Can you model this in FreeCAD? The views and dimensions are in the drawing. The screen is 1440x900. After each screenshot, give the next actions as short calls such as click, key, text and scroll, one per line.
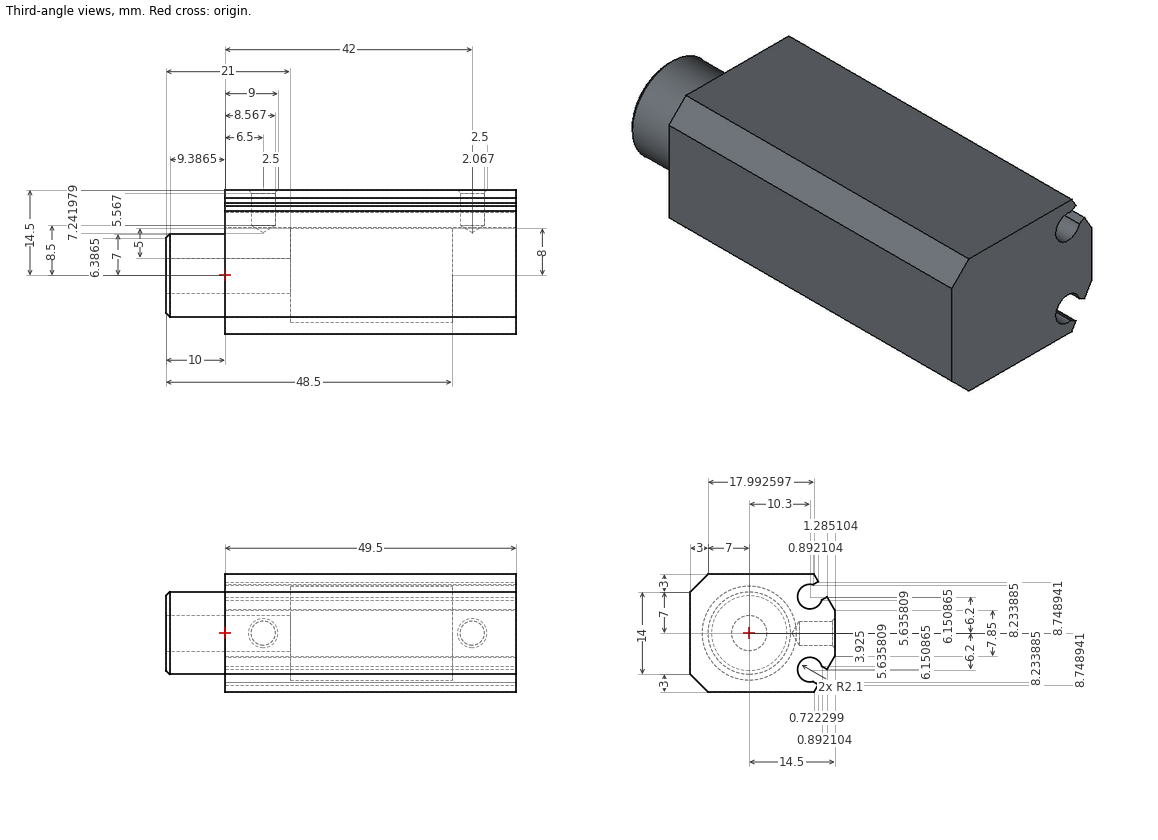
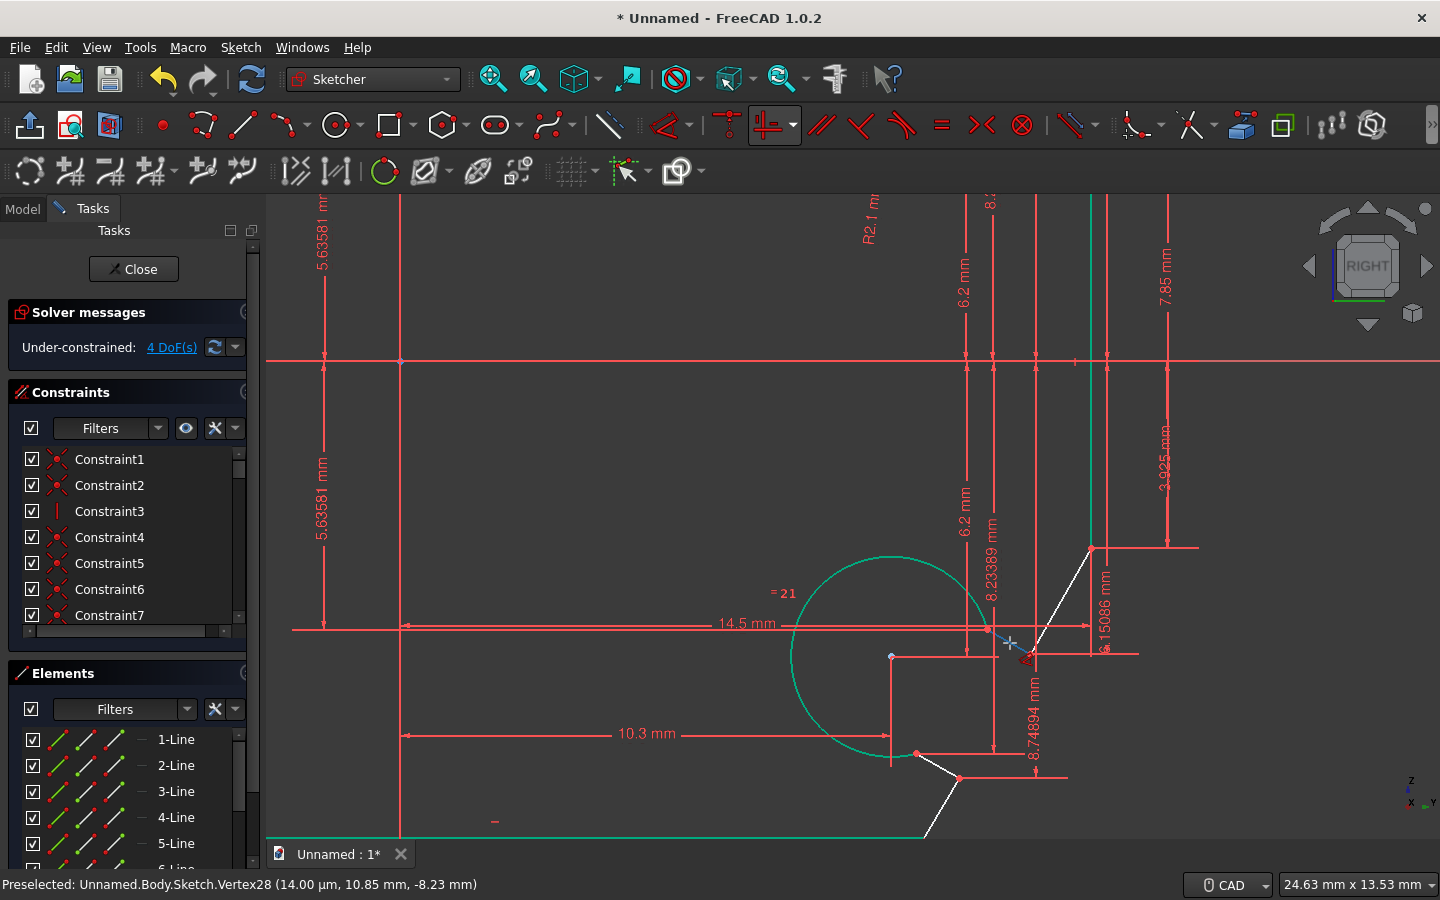
click(1009, 642)
click(1009, 688)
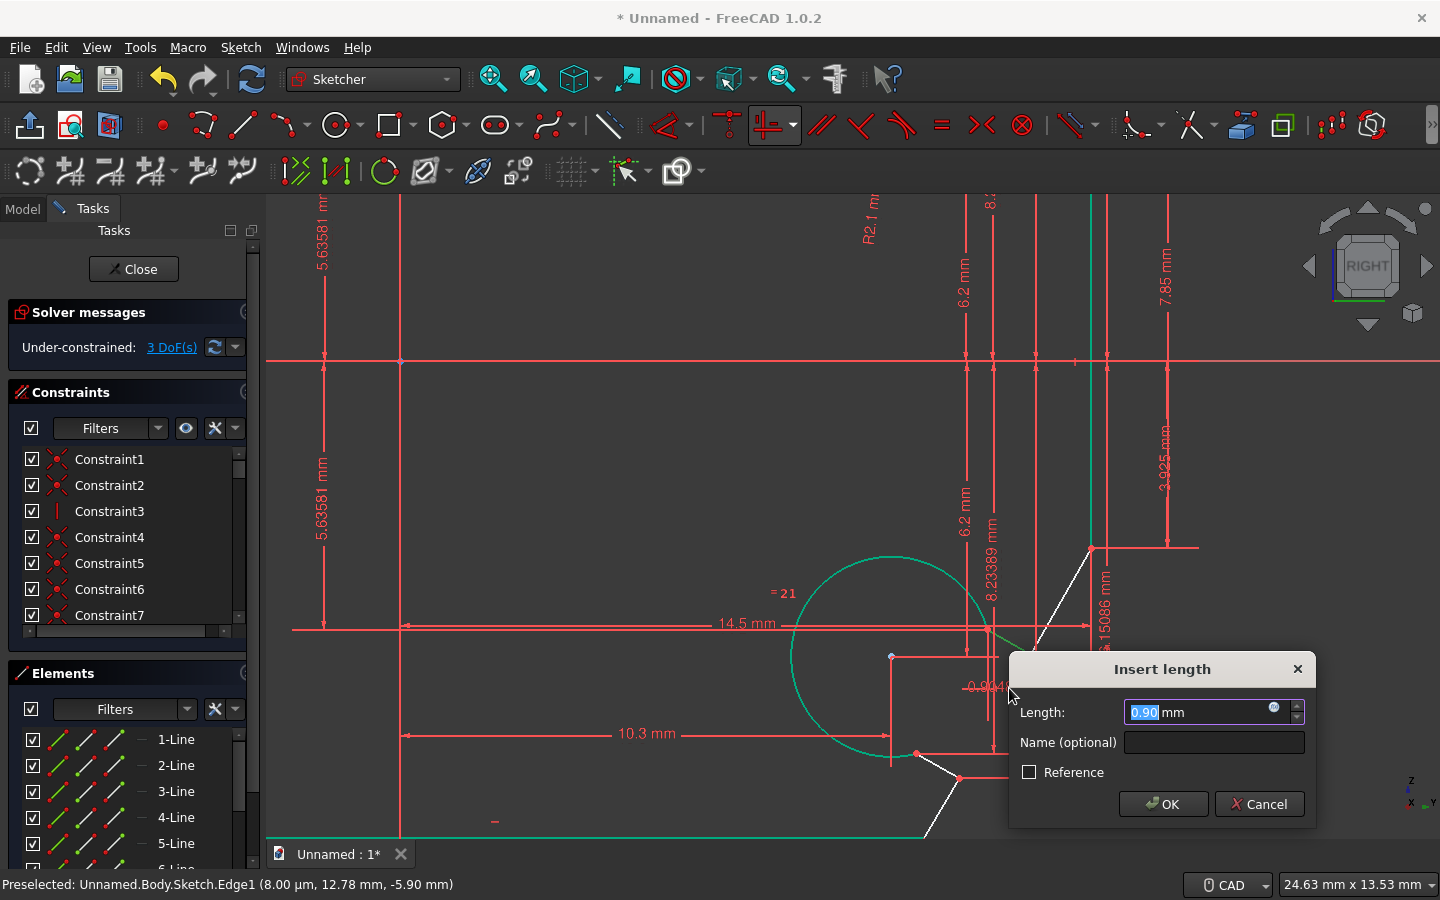
text(0.892104)
key(Return)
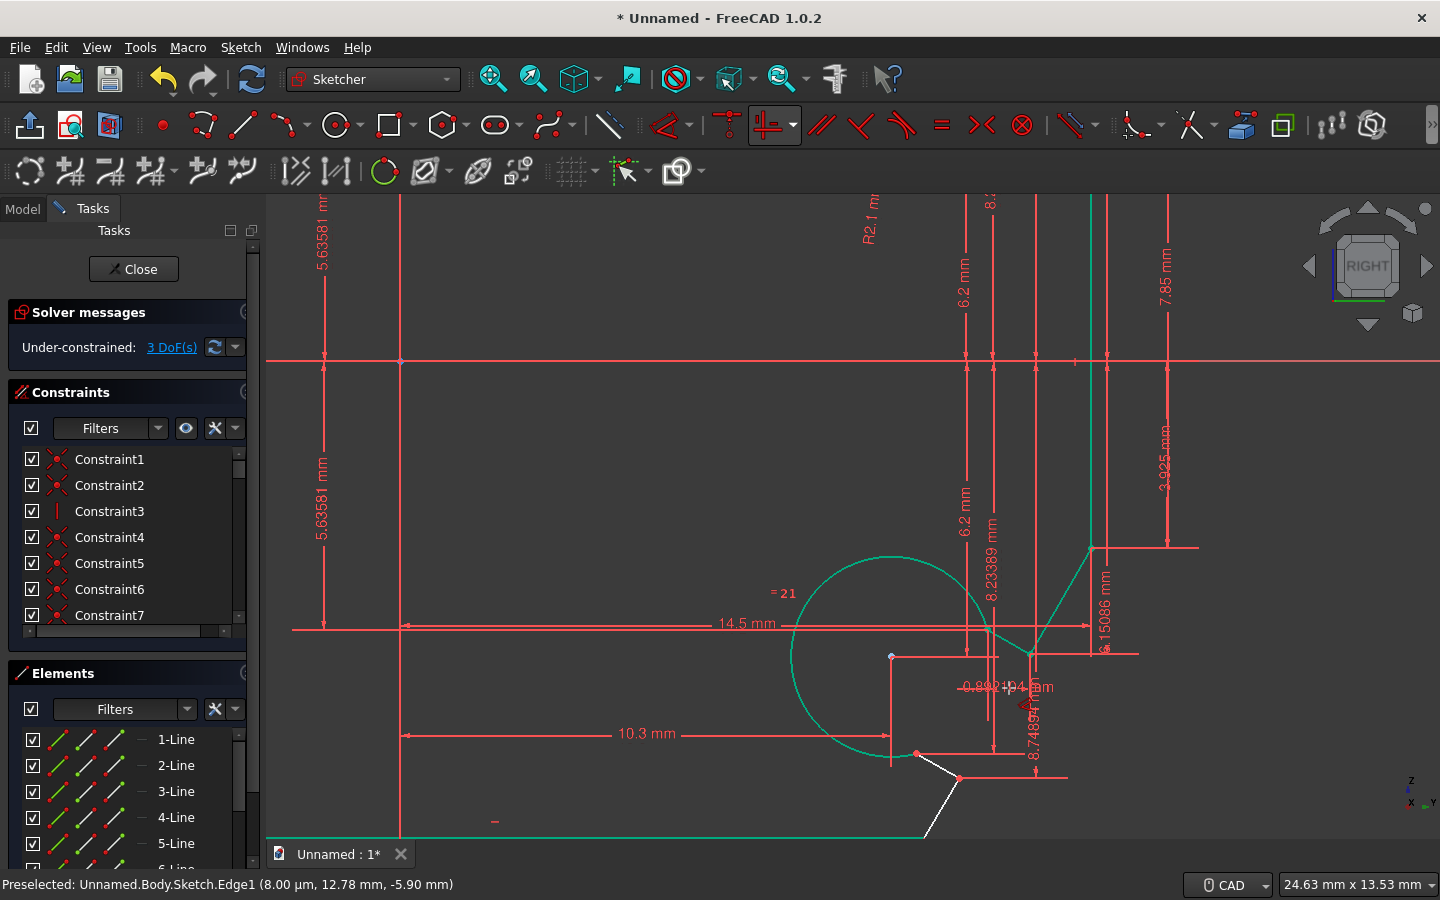
scroll(1010, 643, down, 4)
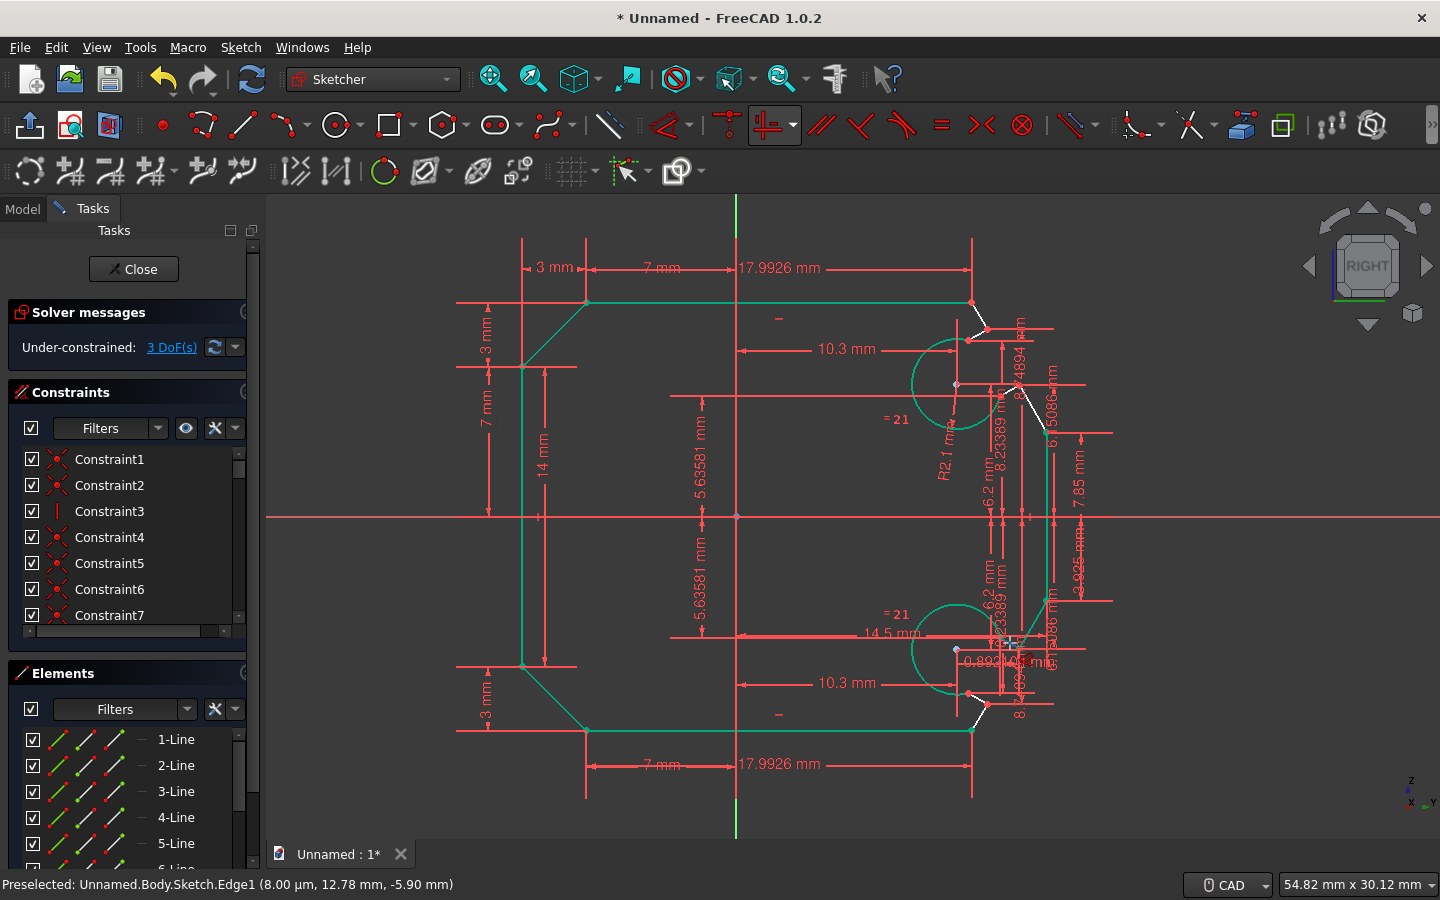
scroll(1039, 418, up, 2)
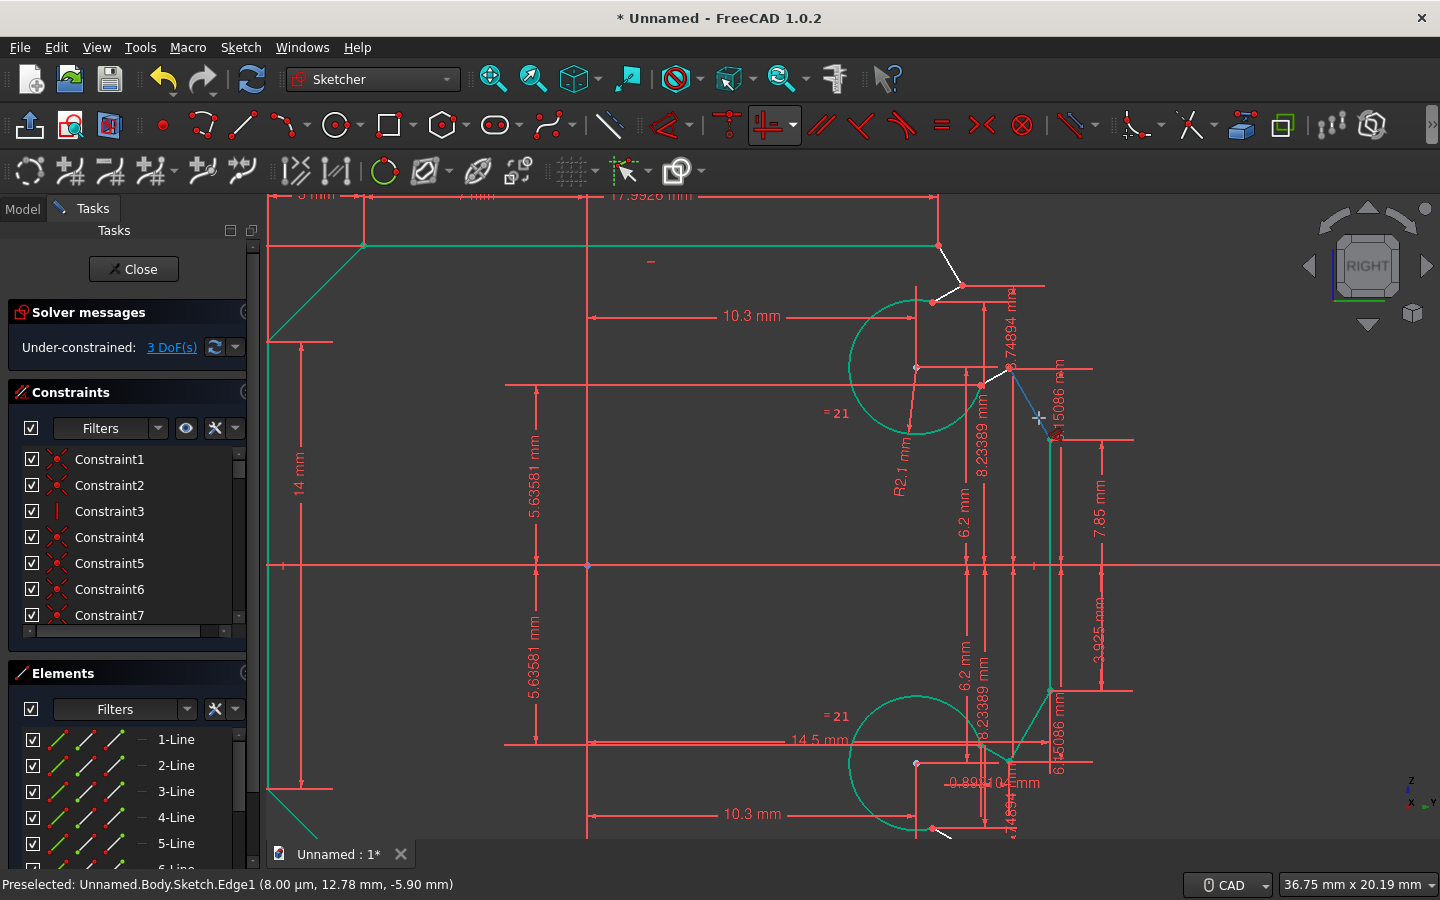
click(1038, 419)
click(1030, 474)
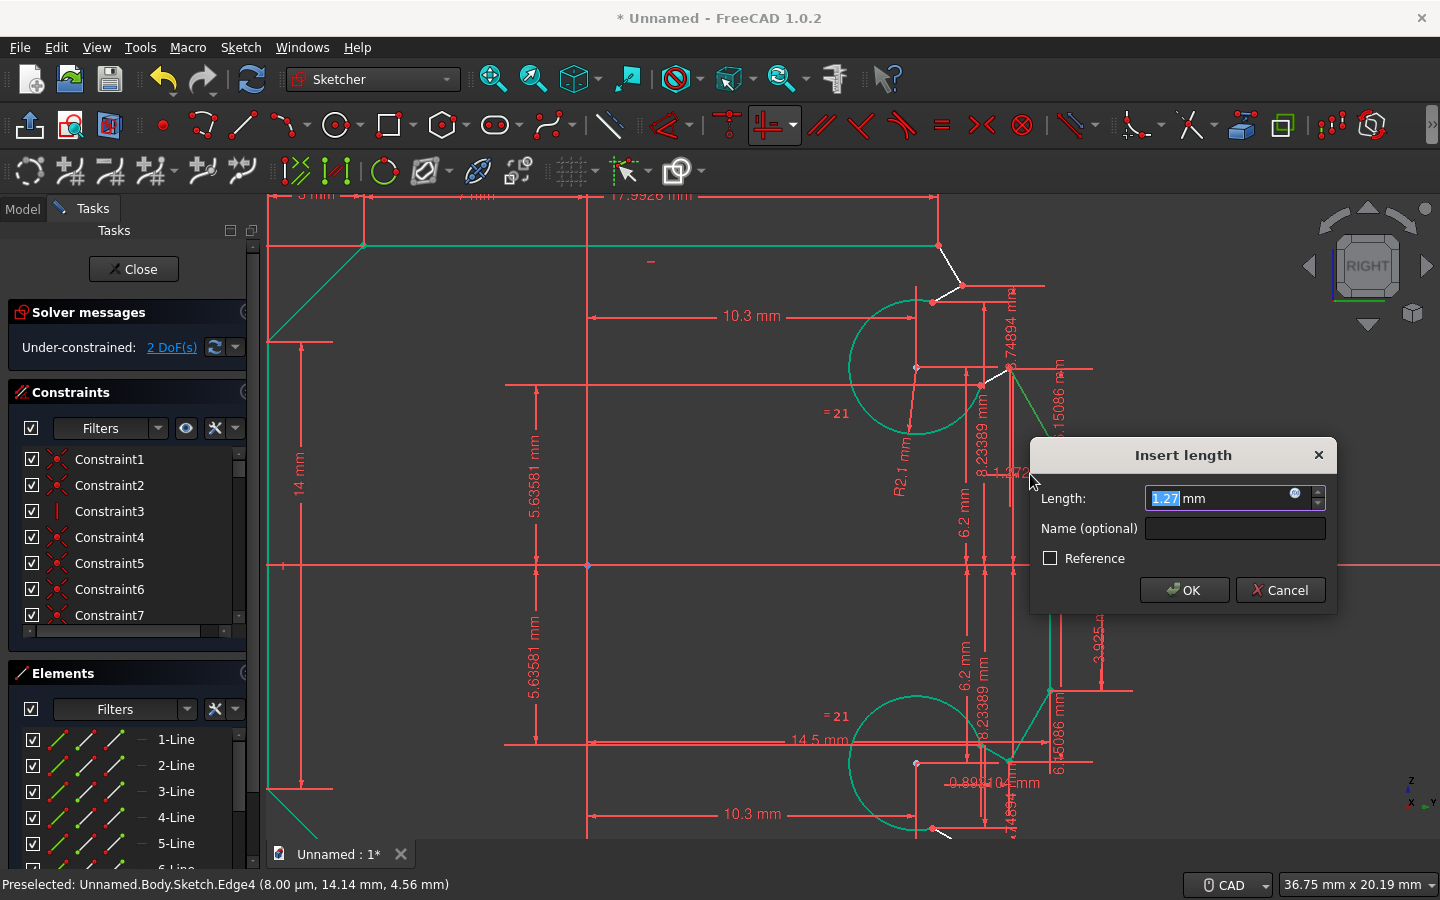
text(1.285104)
key(Return)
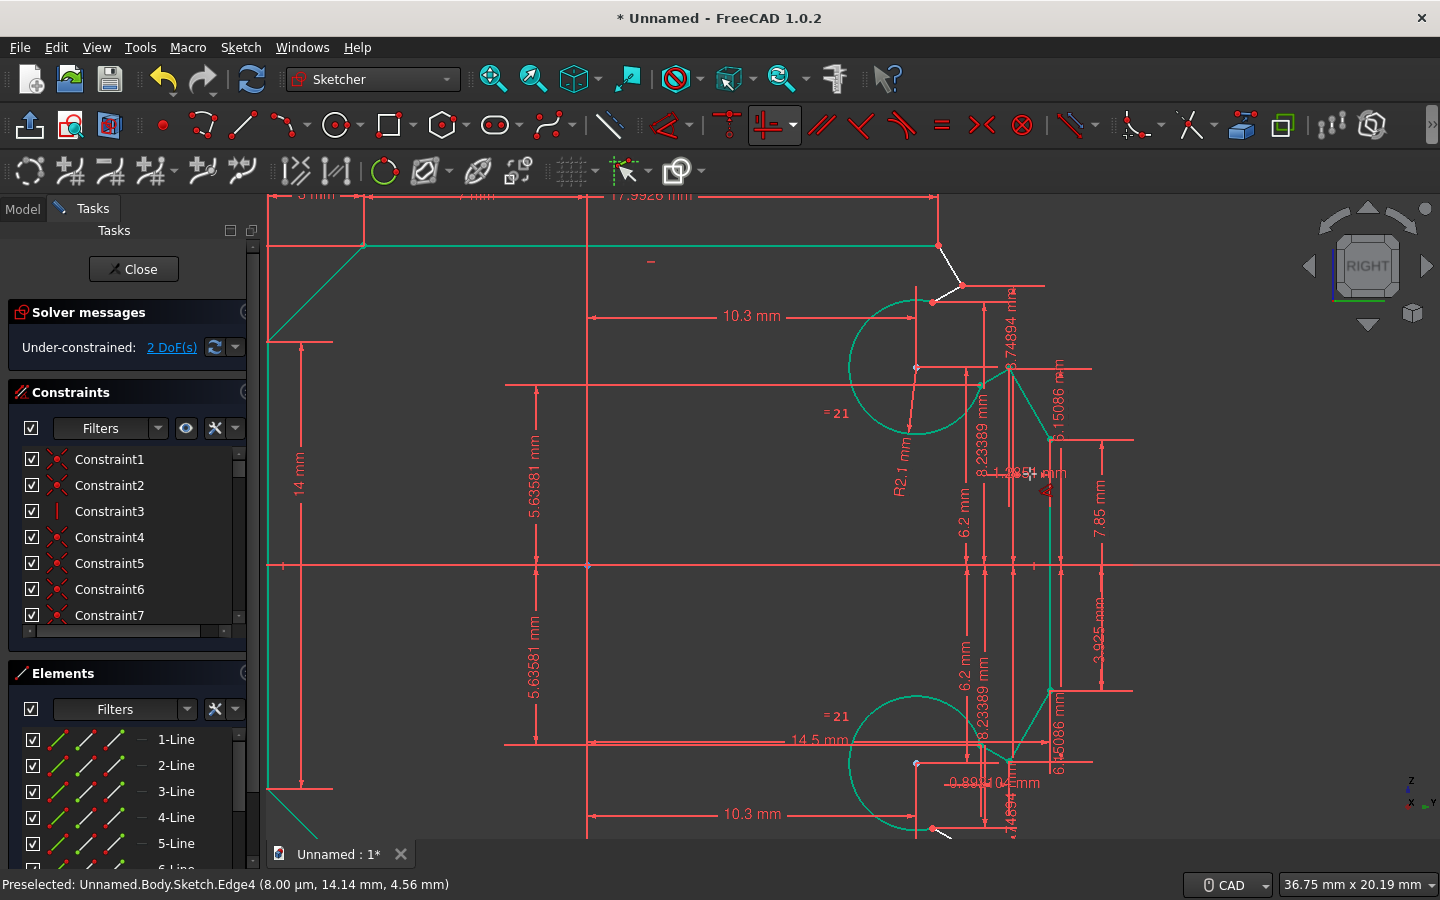
scroll(942, 297, up, 2)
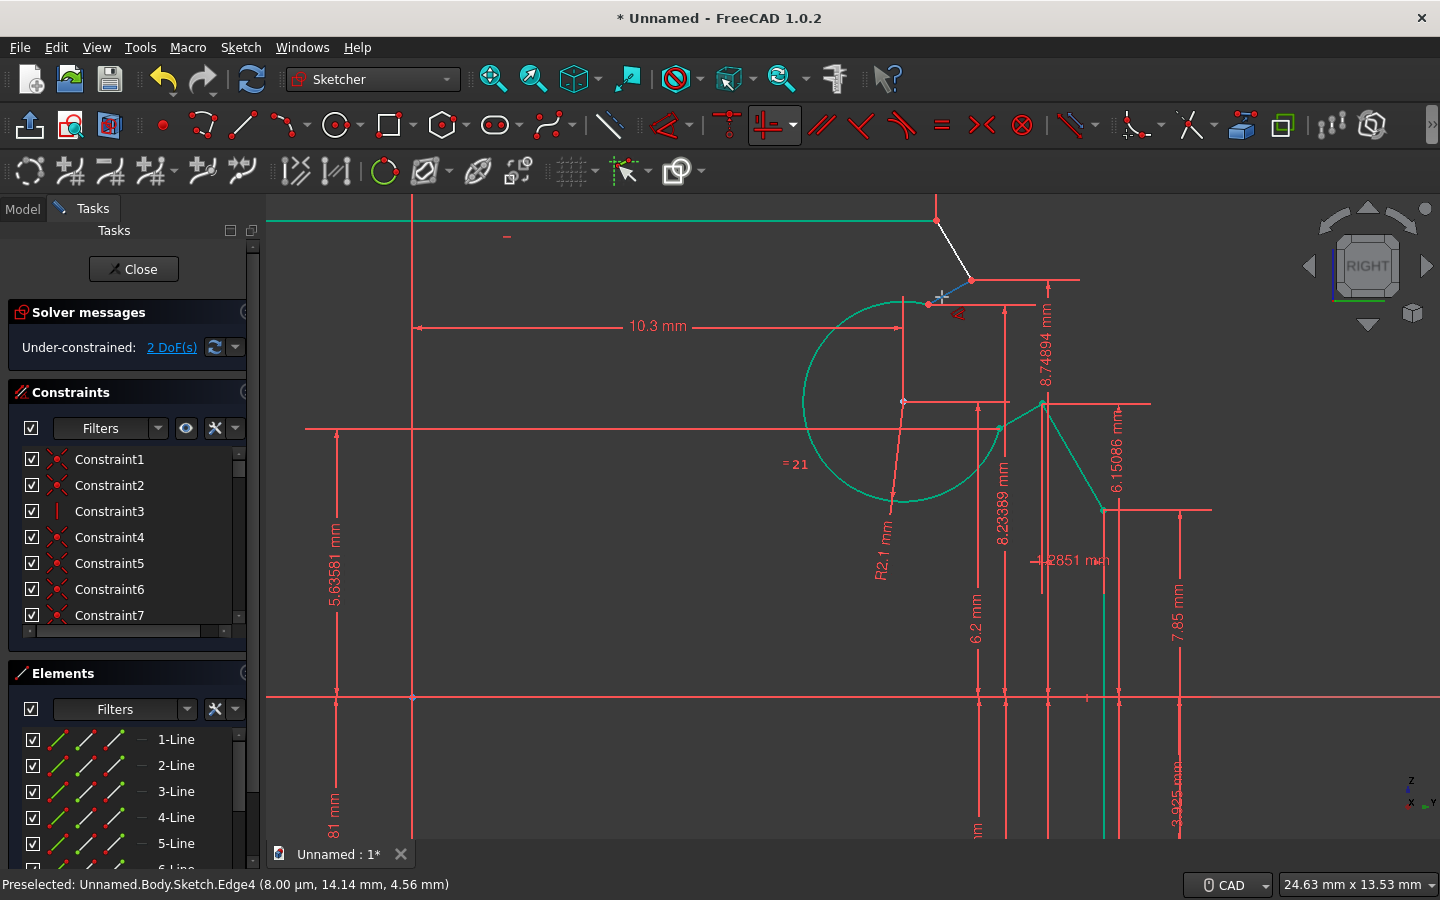
click(941, 297)
click(935, 246)